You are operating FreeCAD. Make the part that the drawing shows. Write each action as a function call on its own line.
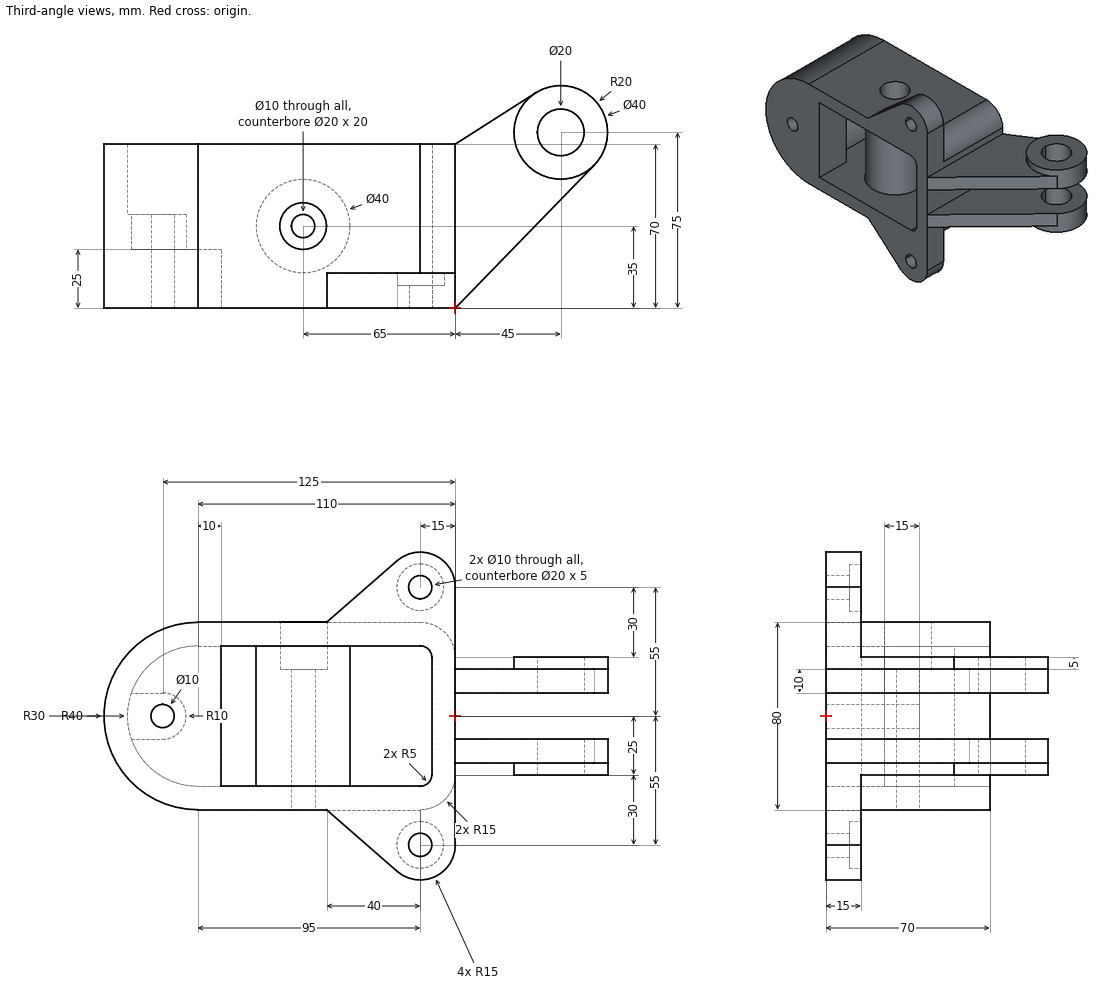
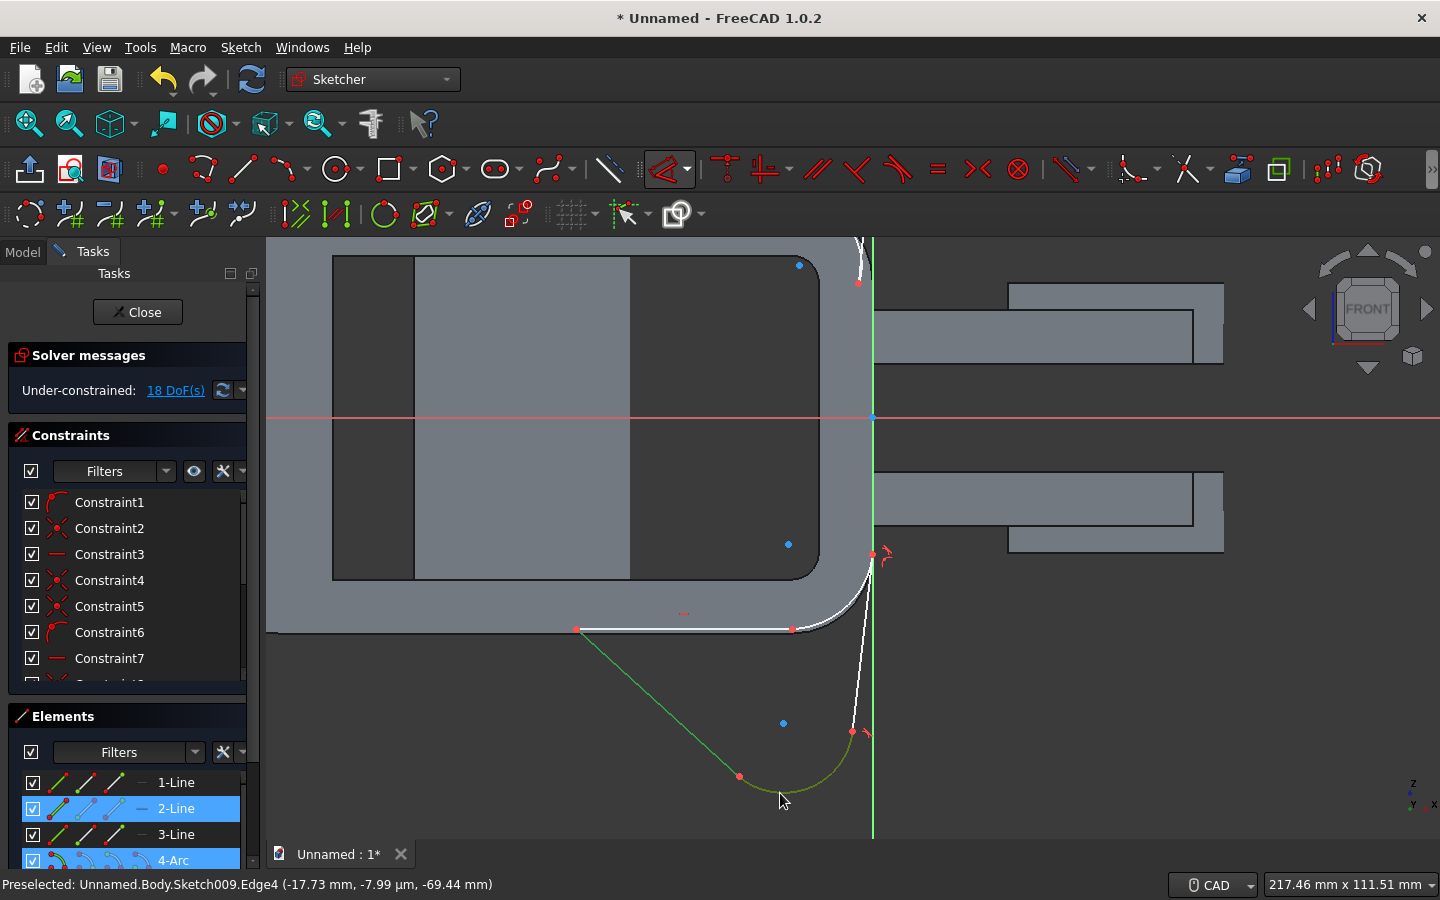
click(898, 170)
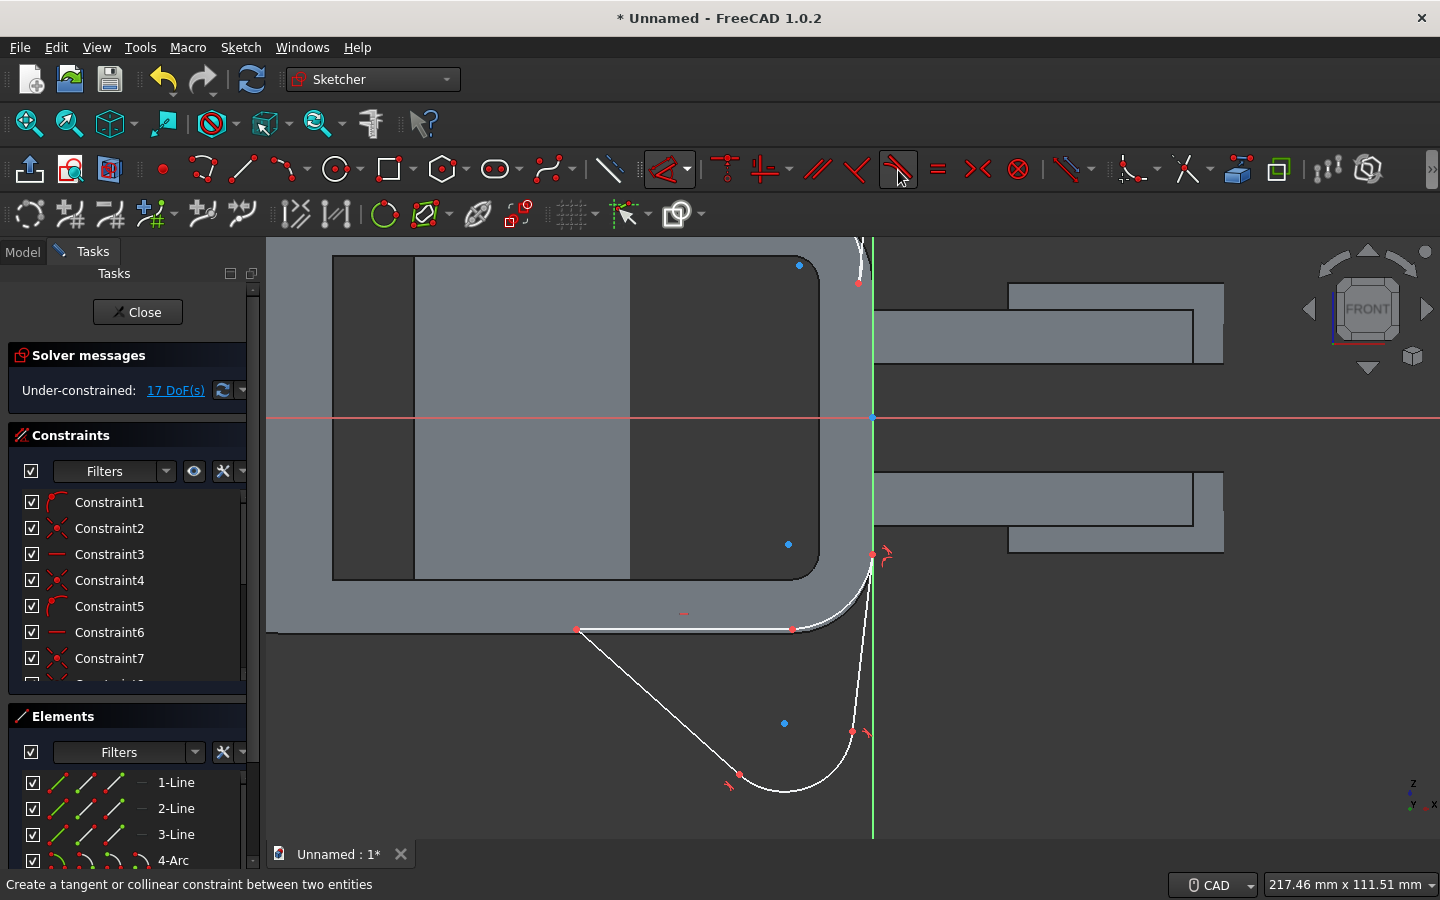
click(641, 629)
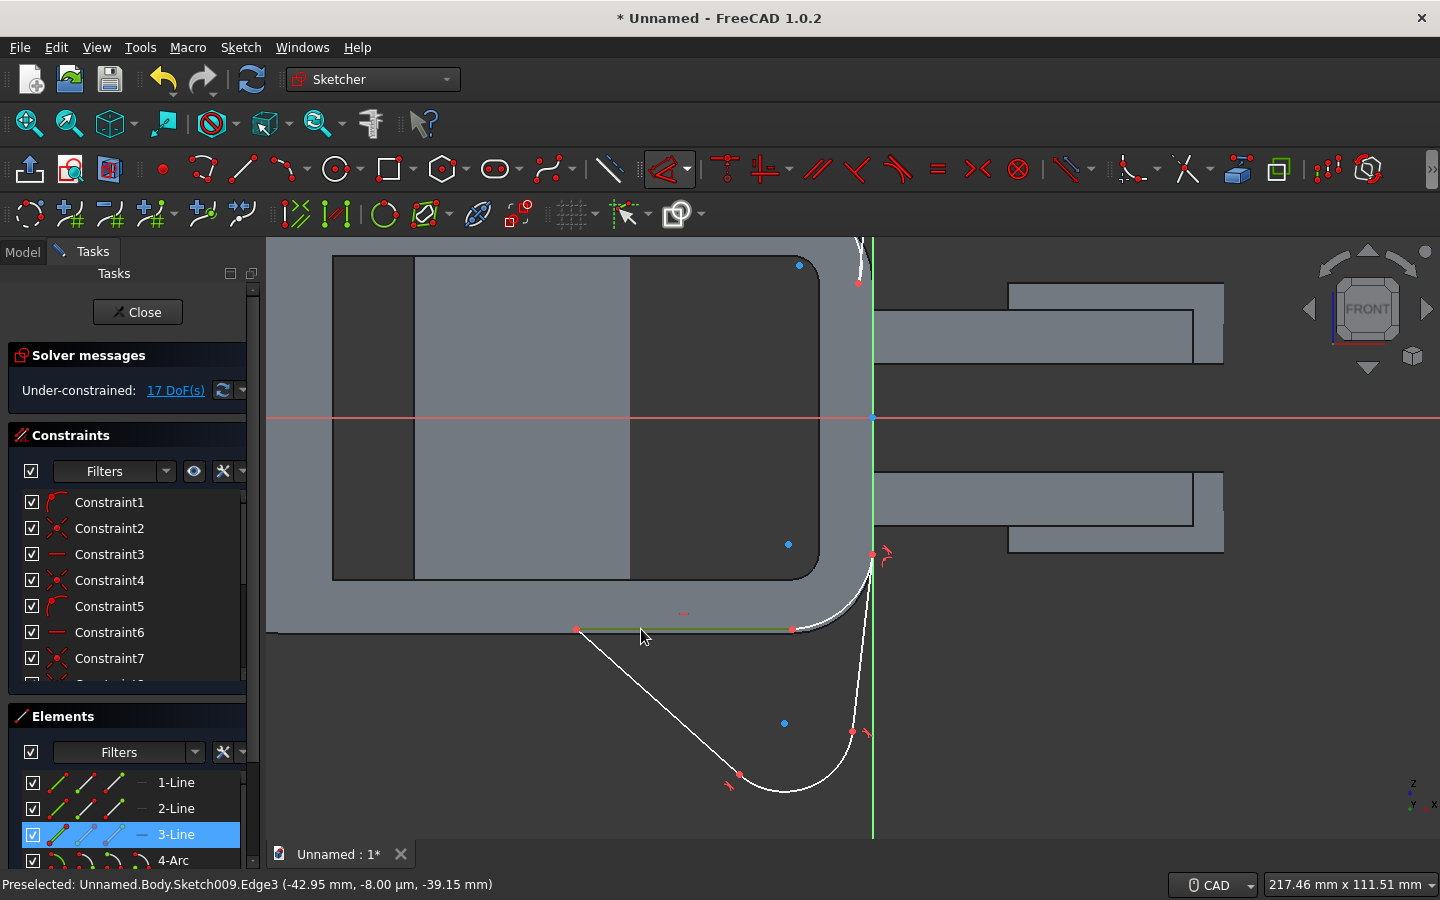
click(827, 620)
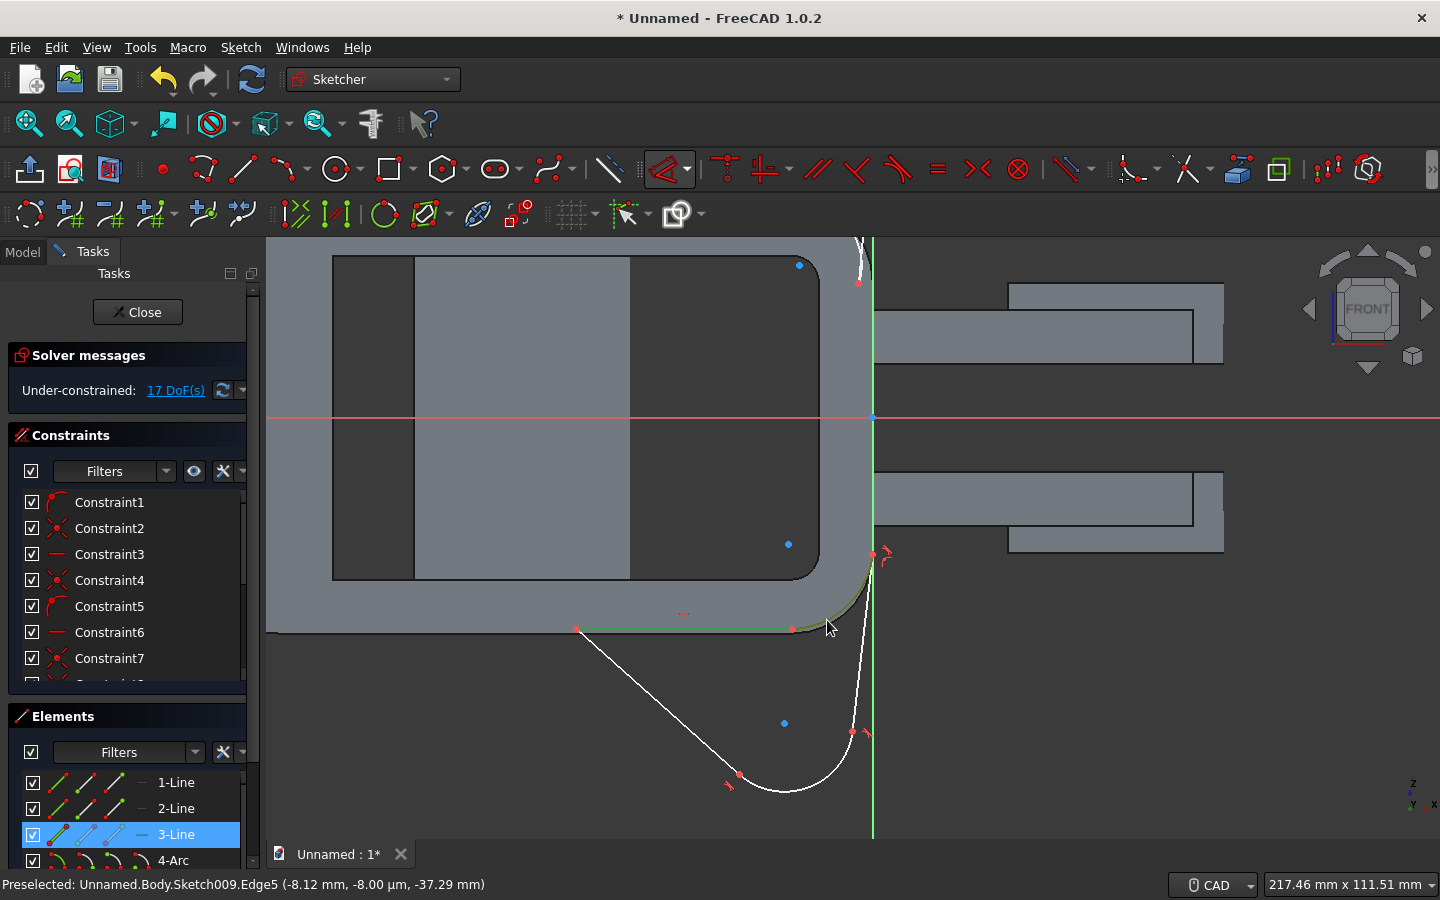
key(t)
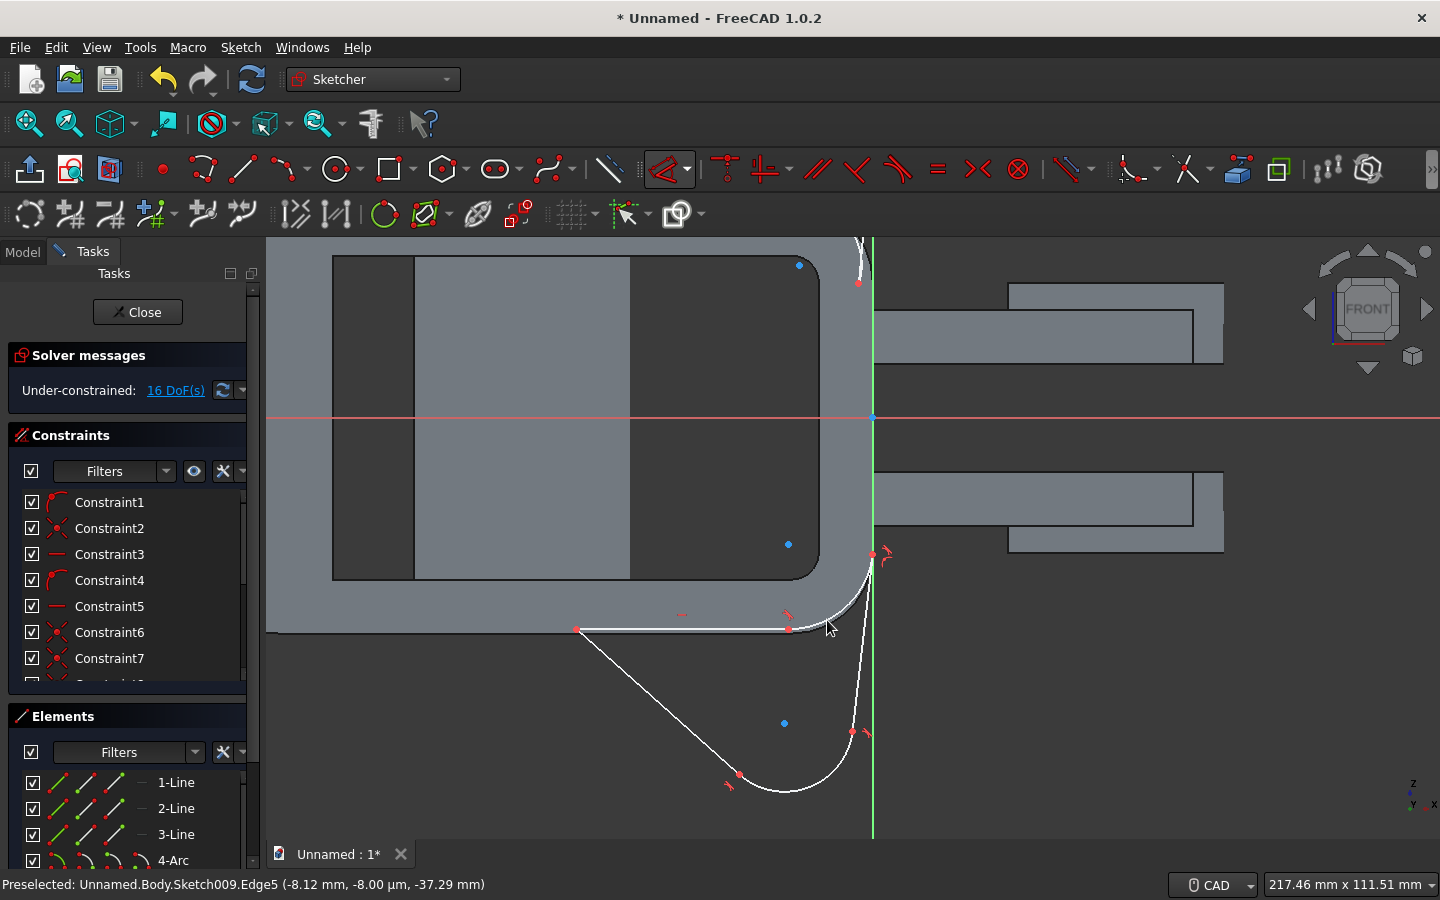
scroll(858, 684, down, 3)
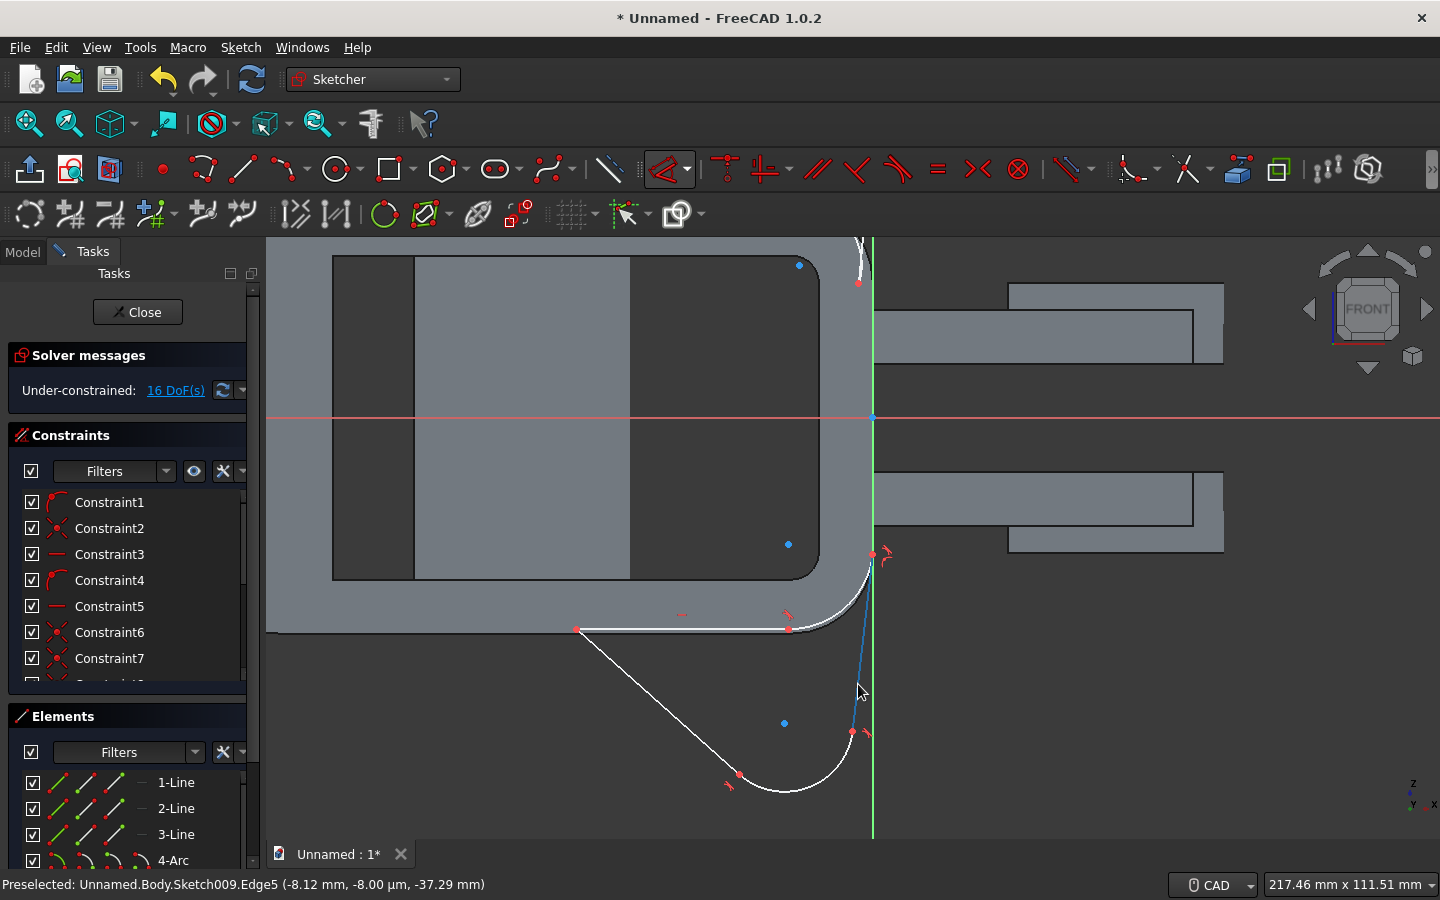
click(865, 394)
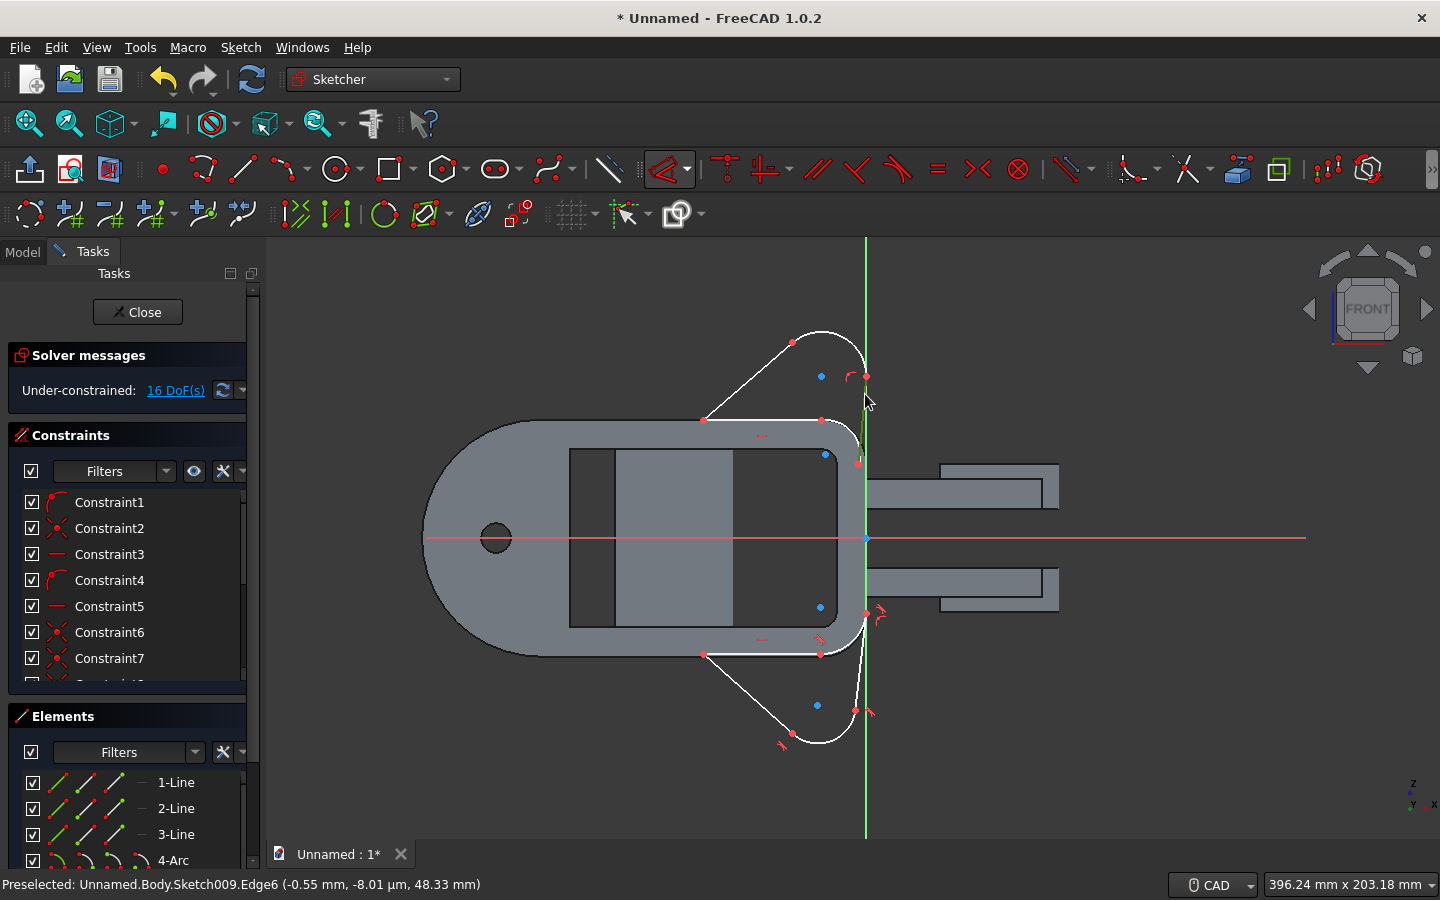
click(842, 424)